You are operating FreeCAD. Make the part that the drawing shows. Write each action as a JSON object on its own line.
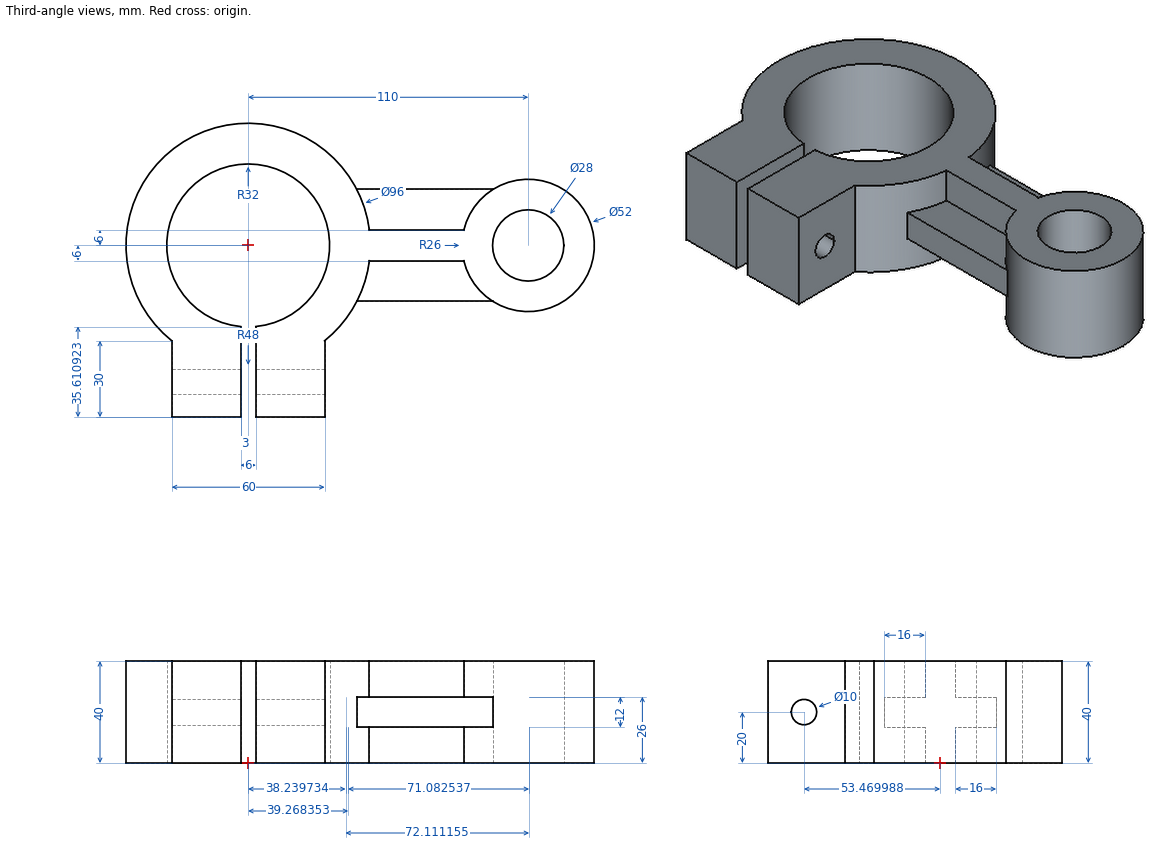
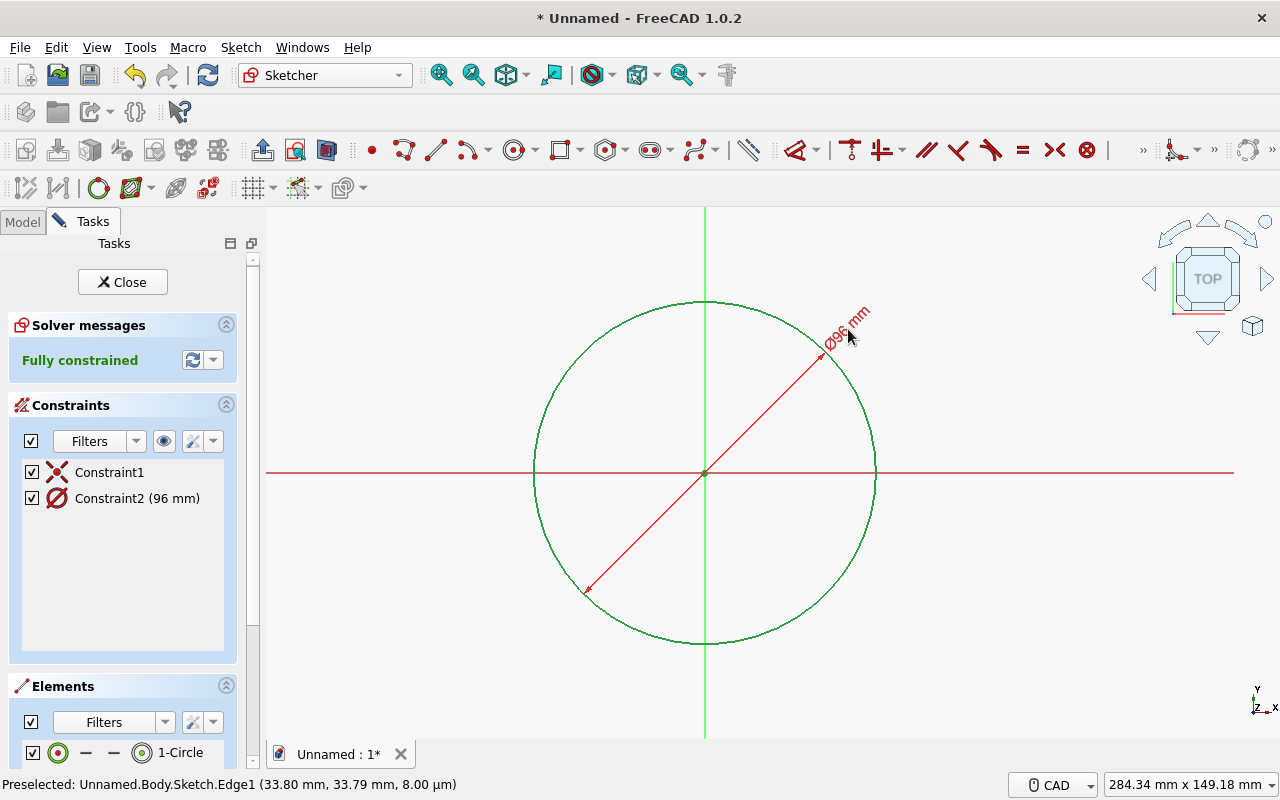
{"action": "left_click", "coordinate": [123, 282]}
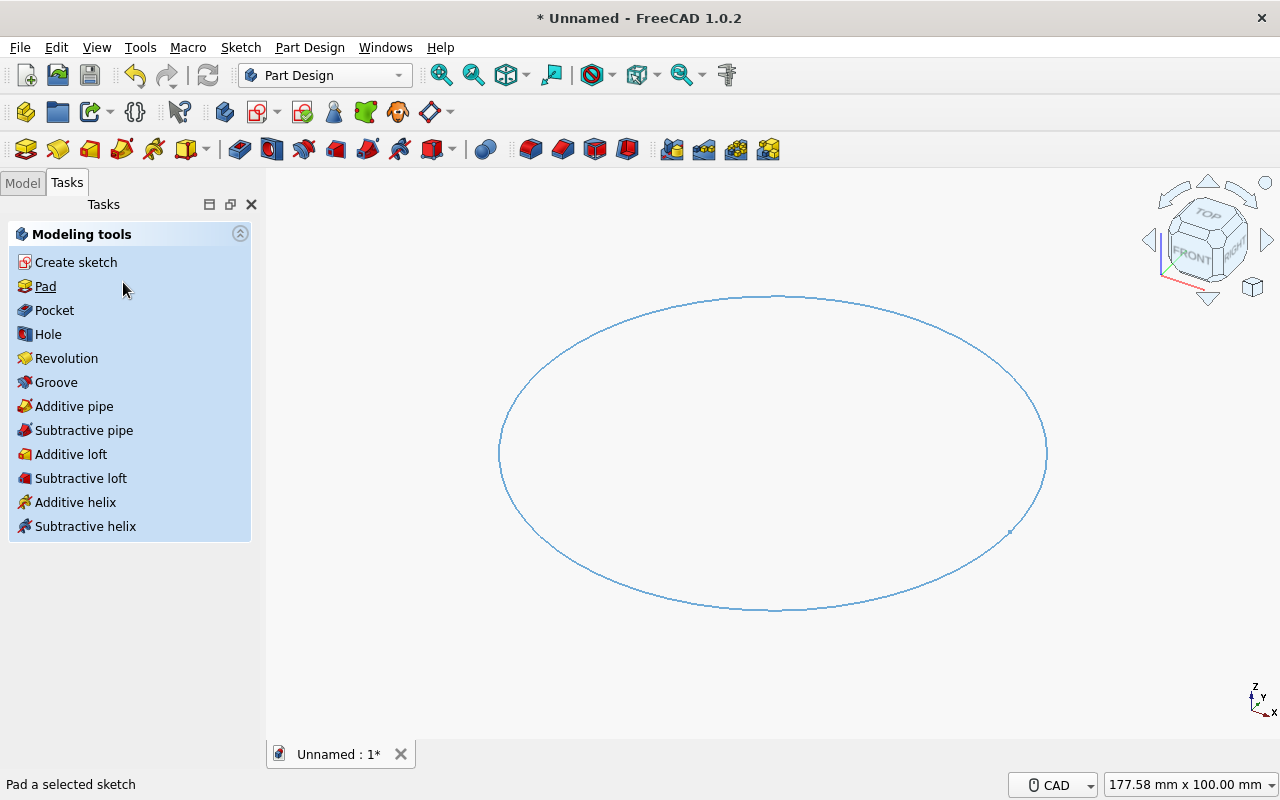
{"action": "left_click", "coordinate": [26, 150]}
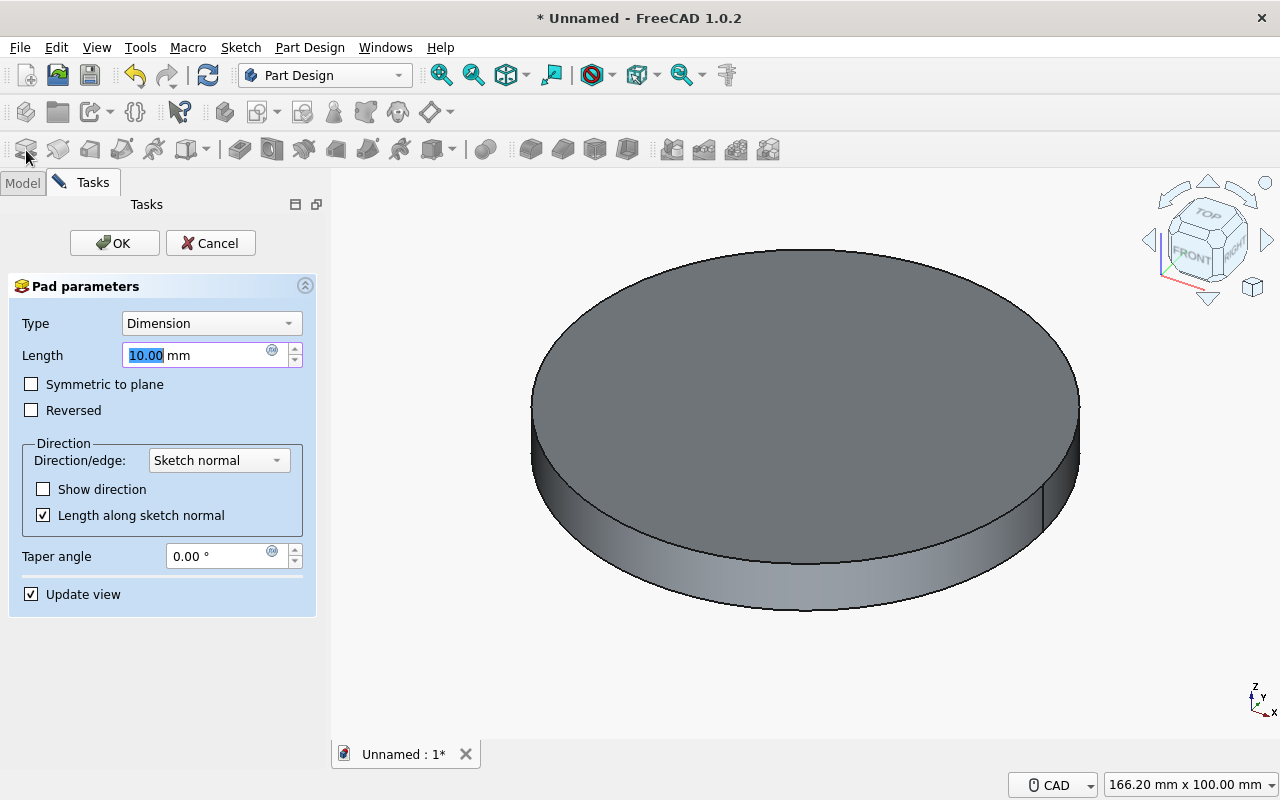
{"action": "type", "text": "40"}
{"action": "key", "text": "Tab"}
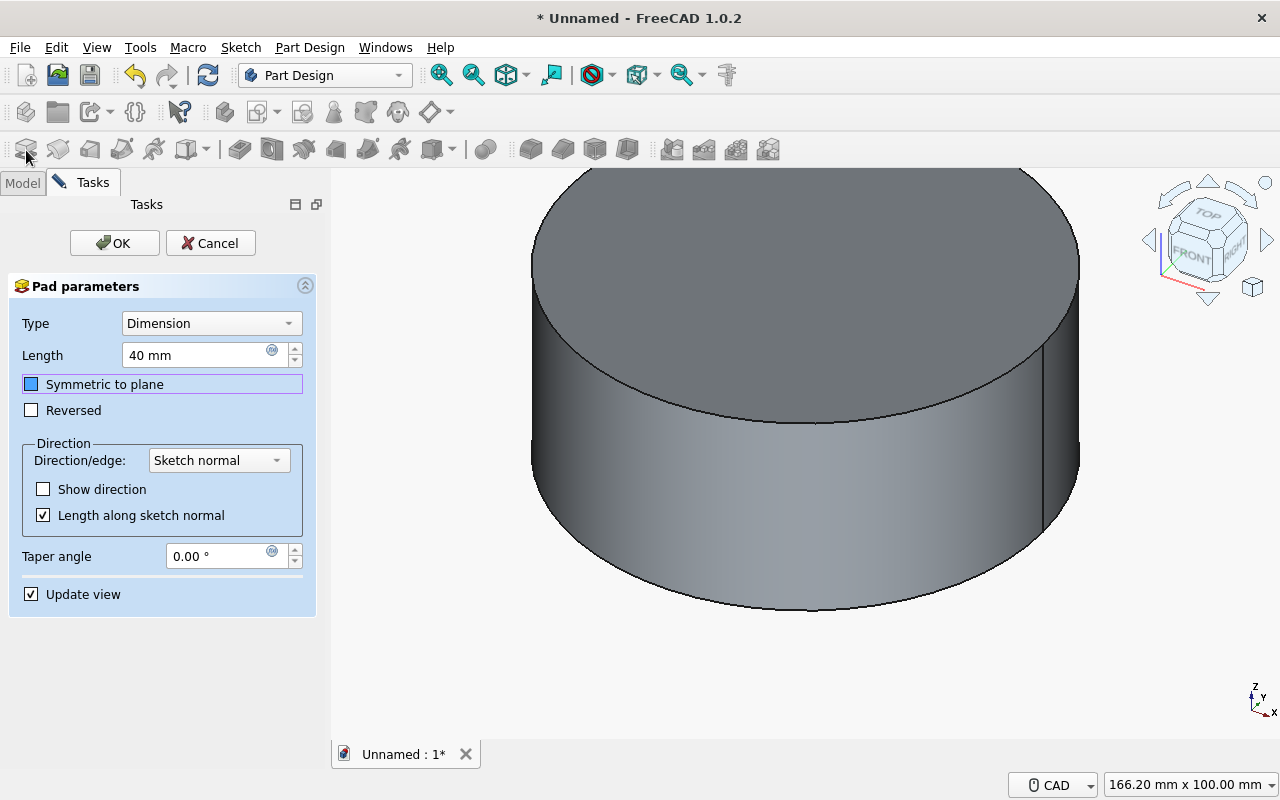
{"action": "left_click", "coordinate": [115, 243]}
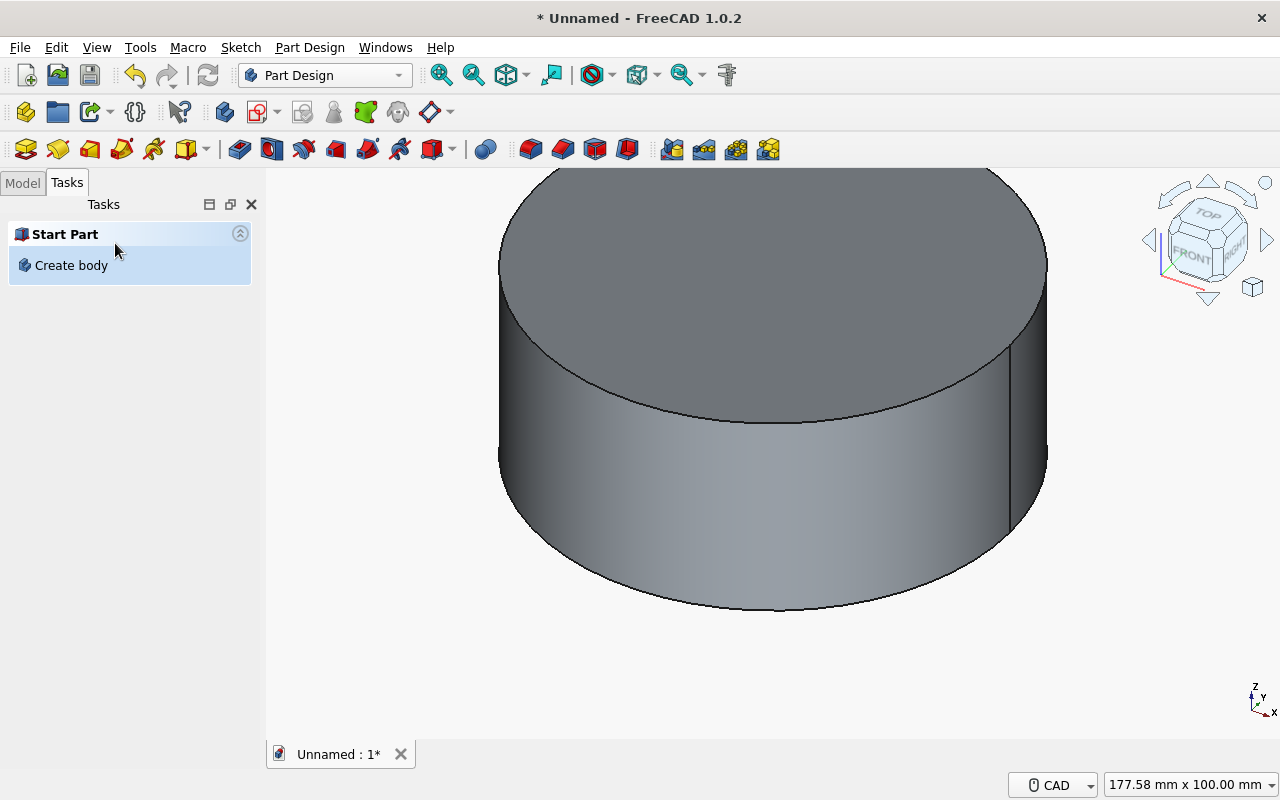
{"action": "left_click", "coordinate": [442, 76]}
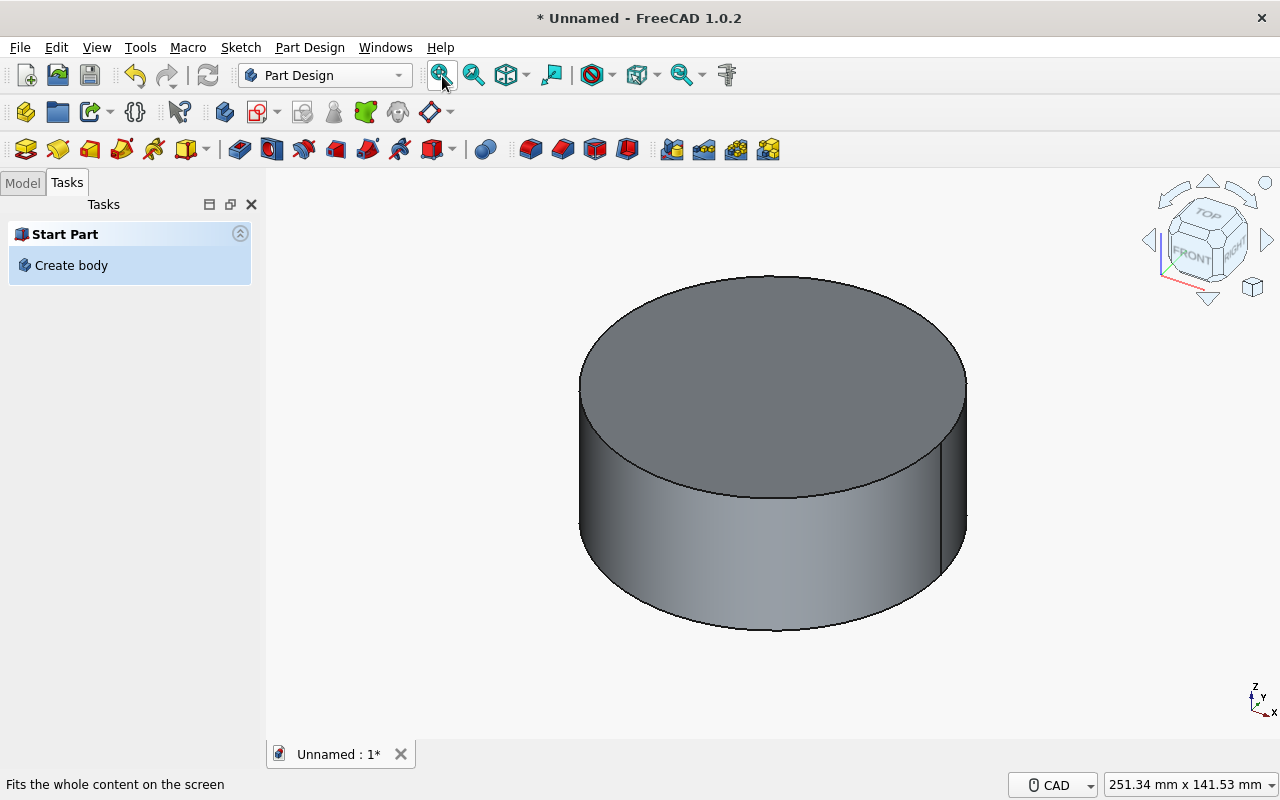
{"action": "key", "text": "5"}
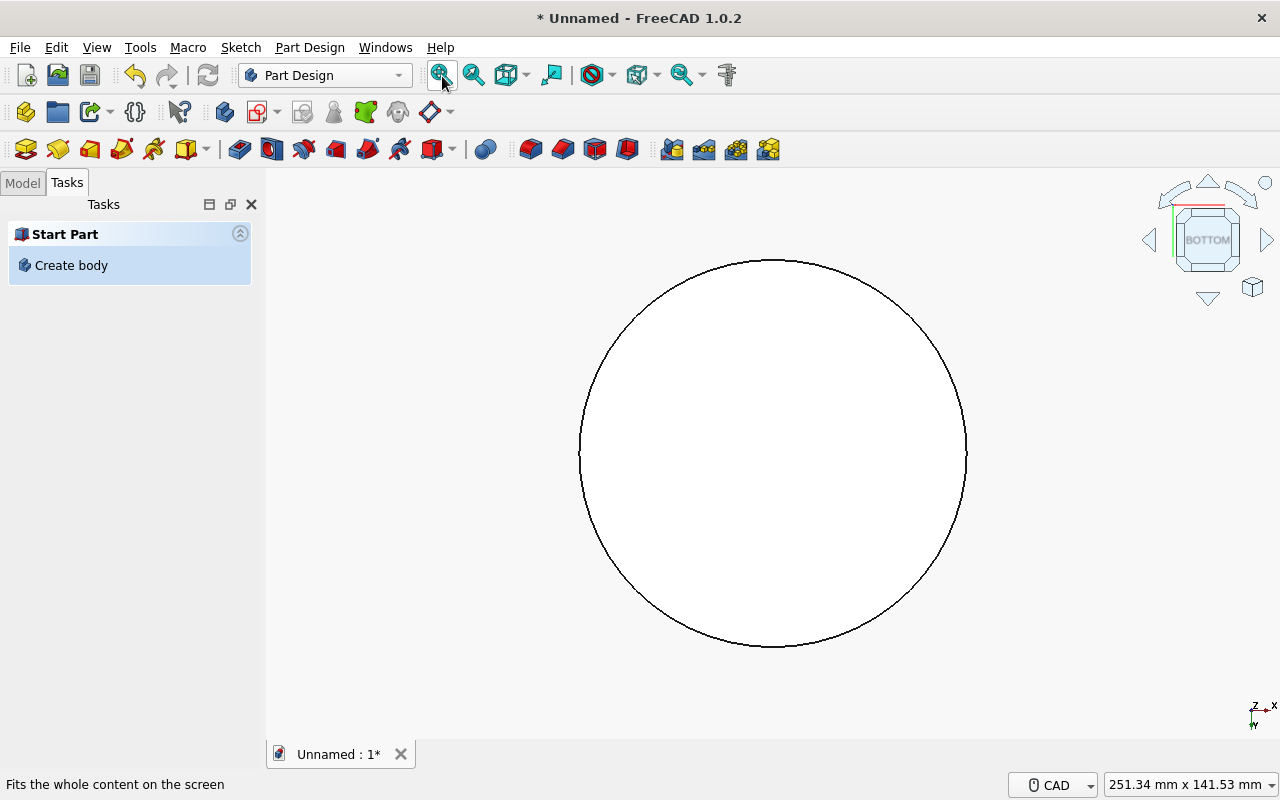
{"action": "left_click", "coordinate": [773, 452]}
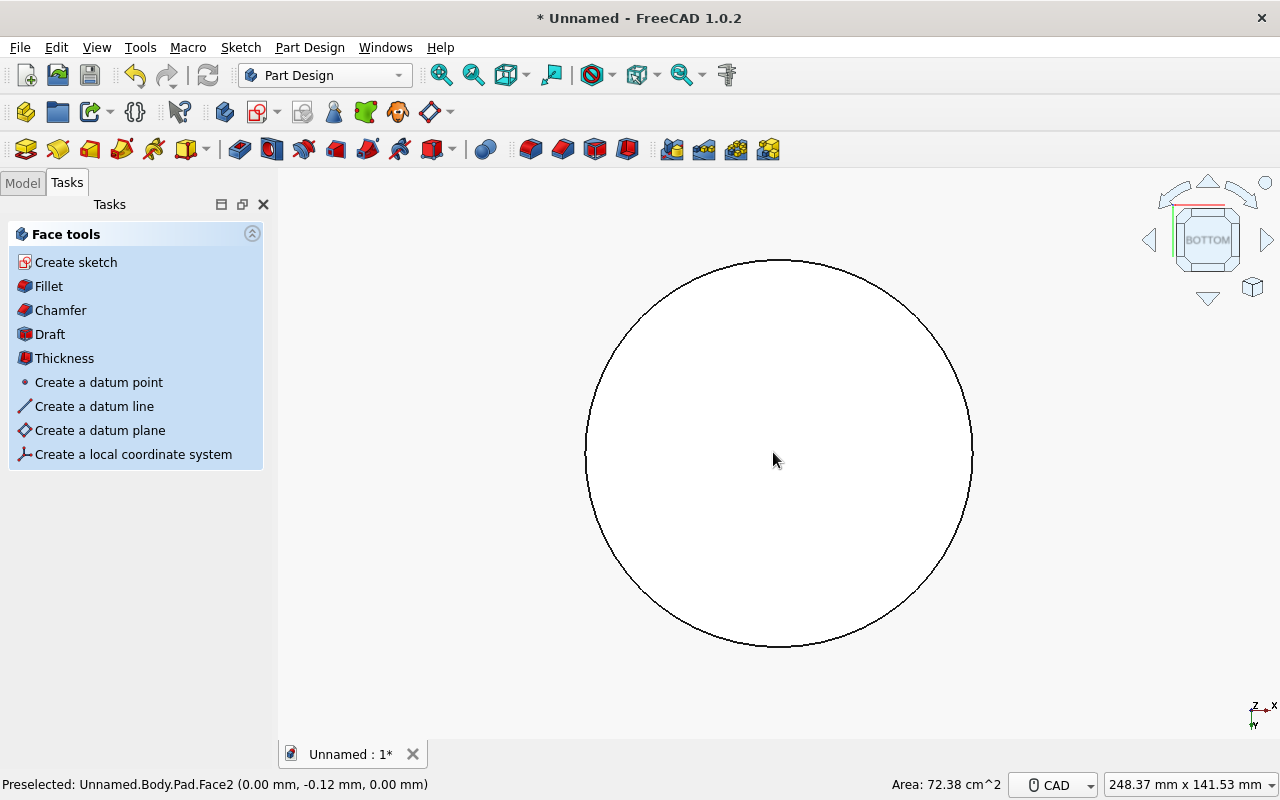
{"action": "left_click", "coordinate": [258, 112]}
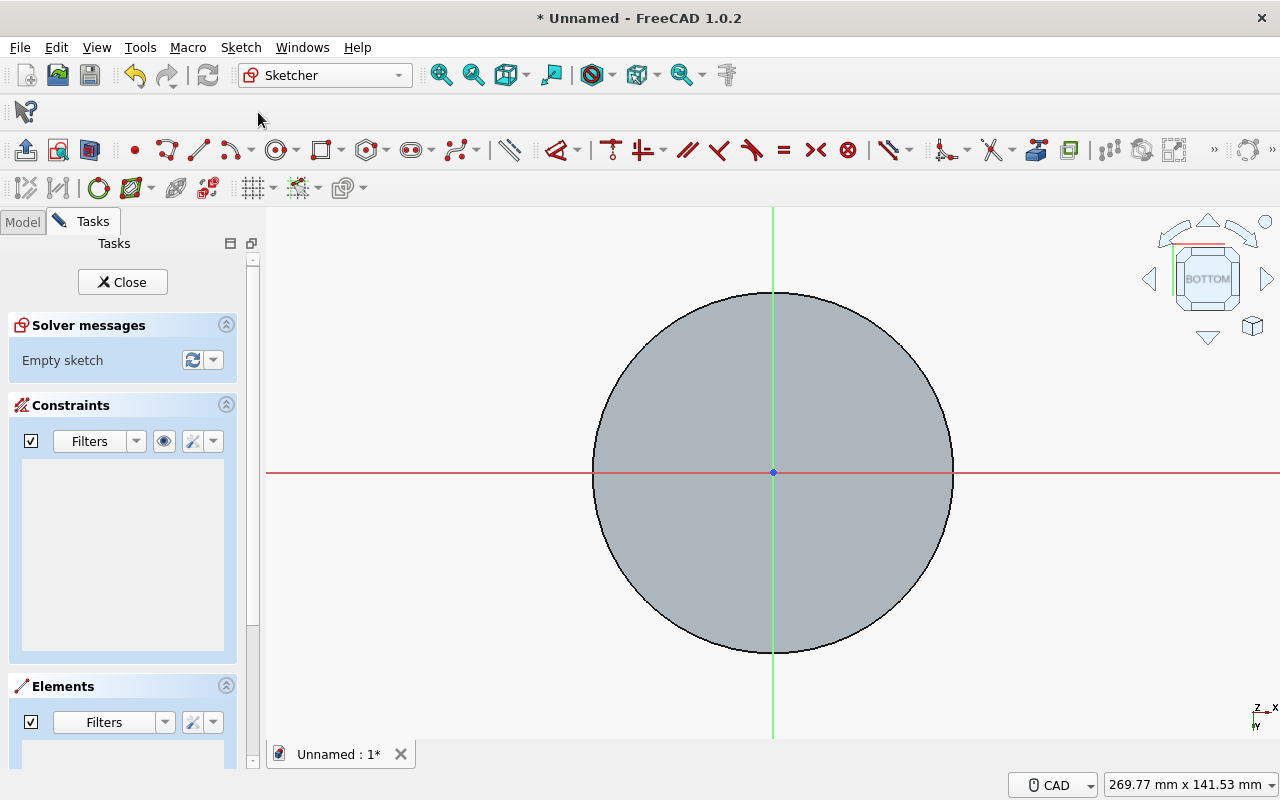
{"action": "scroll", "coordinate": [395, 711], "scroll_direction": "down", "scroll_amount": 1}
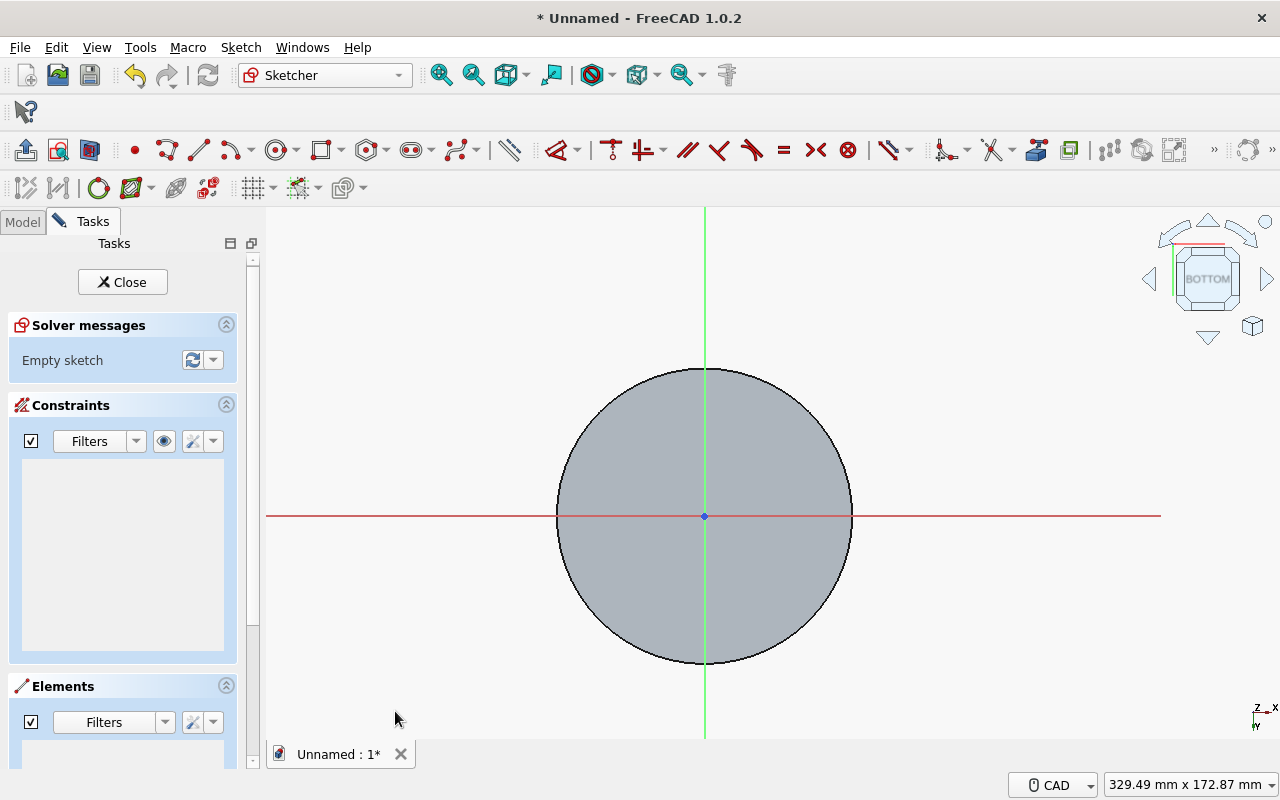
{"action": "scroll", "coordinate": [705, 289], "scroll_direction": "up", "scroll_amount": 2}